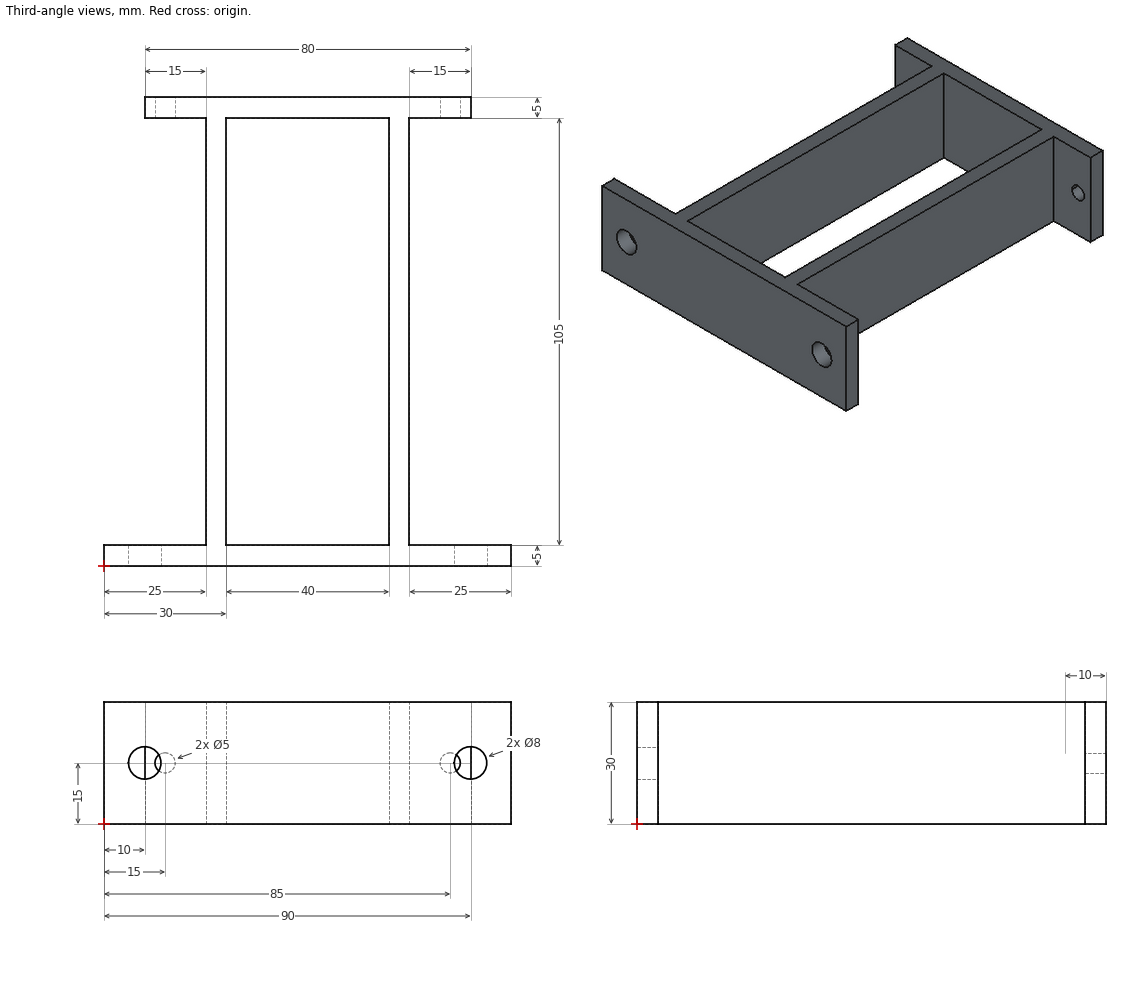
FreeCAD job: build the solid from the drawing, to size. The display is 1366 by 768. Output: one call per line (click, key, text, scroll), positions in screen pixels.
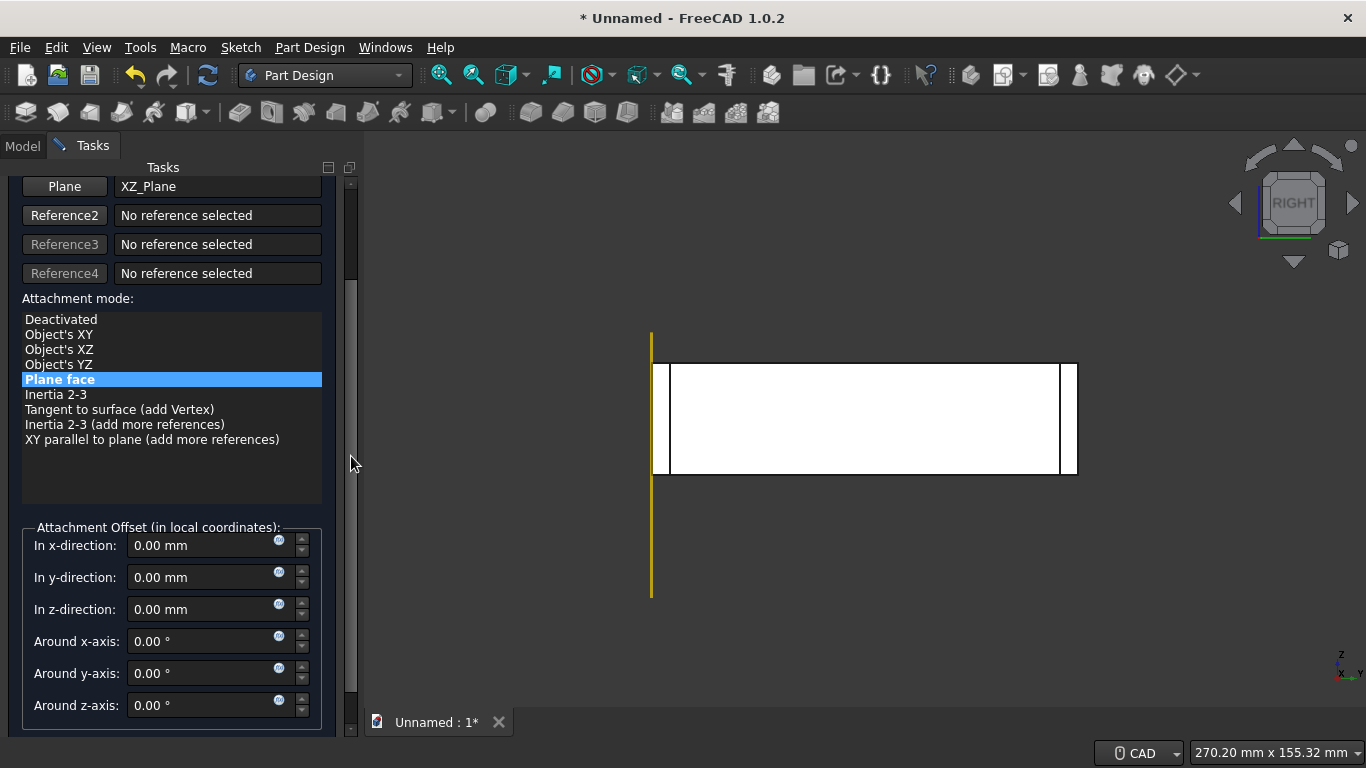
triple_click(210, 609)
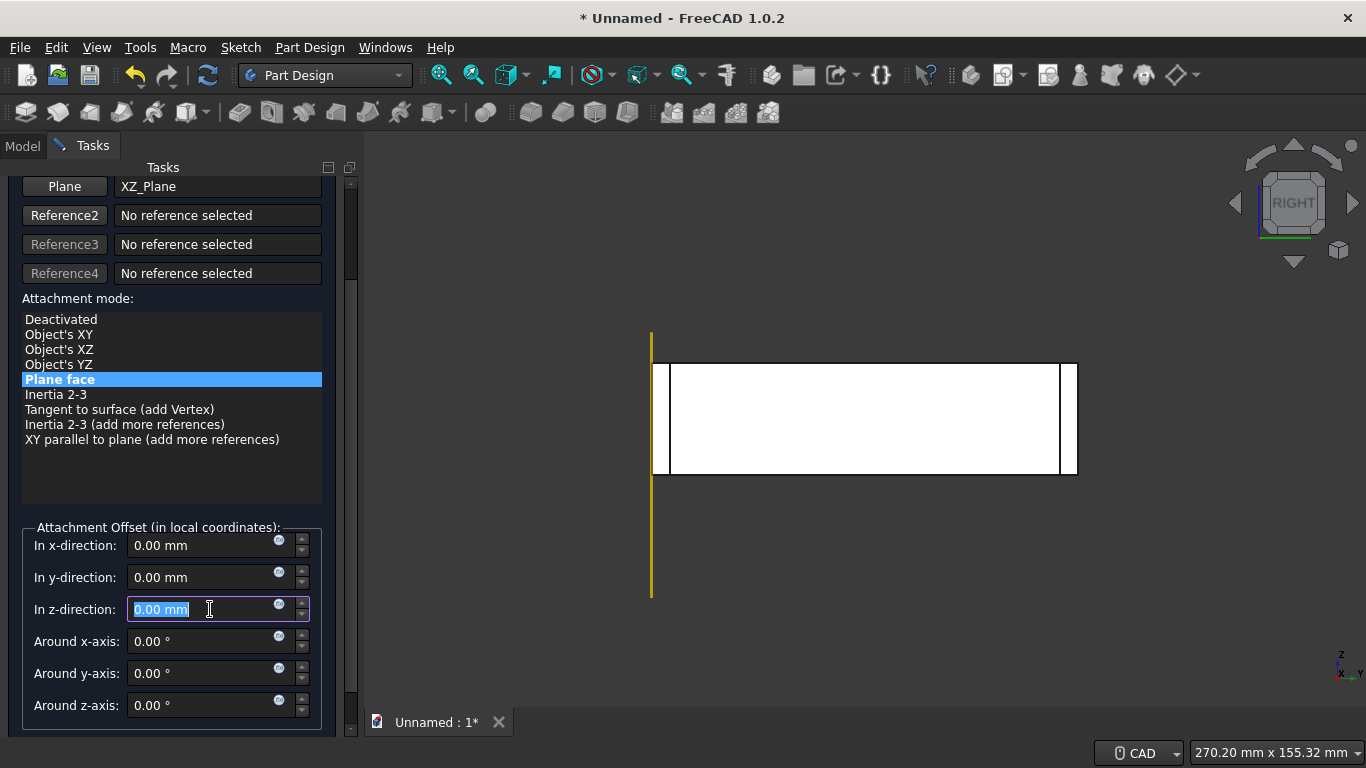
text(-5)
key(Tab)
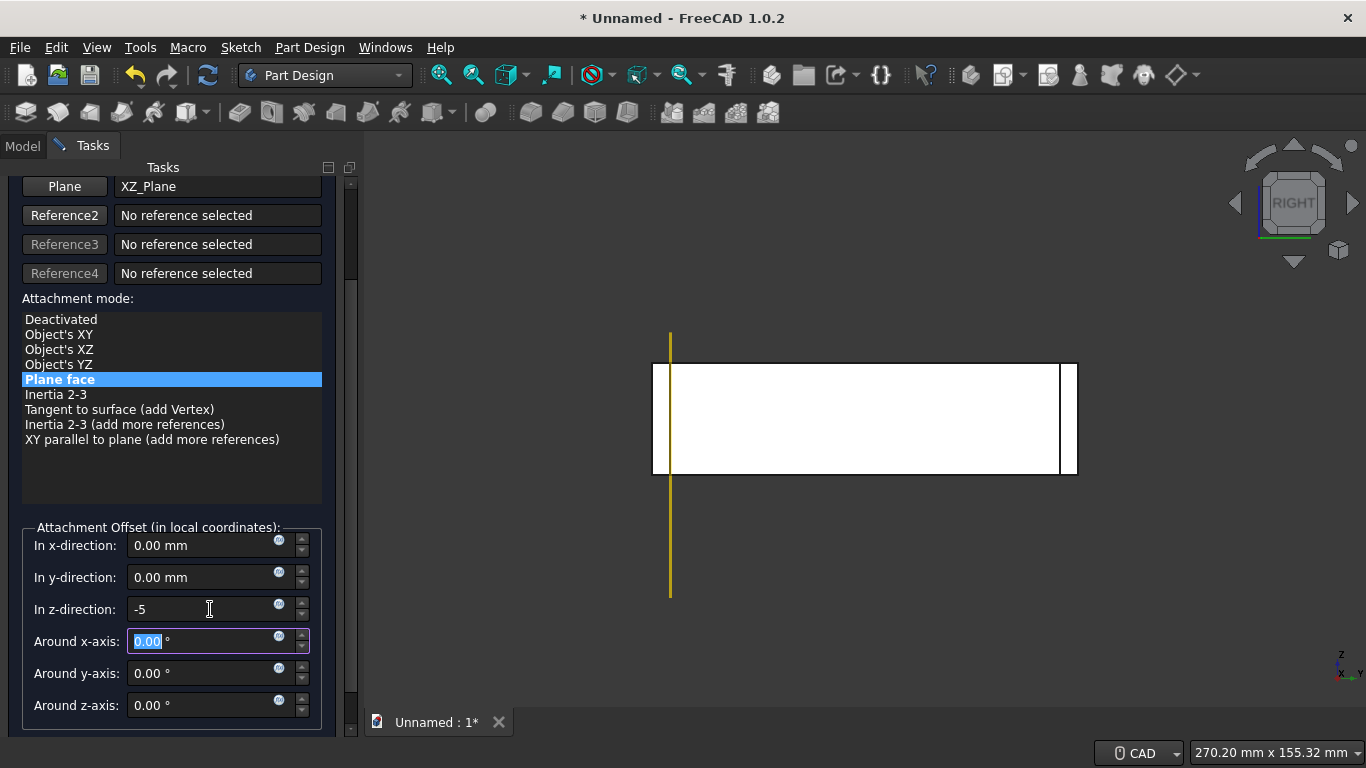
scroll(351, 456, up, 3)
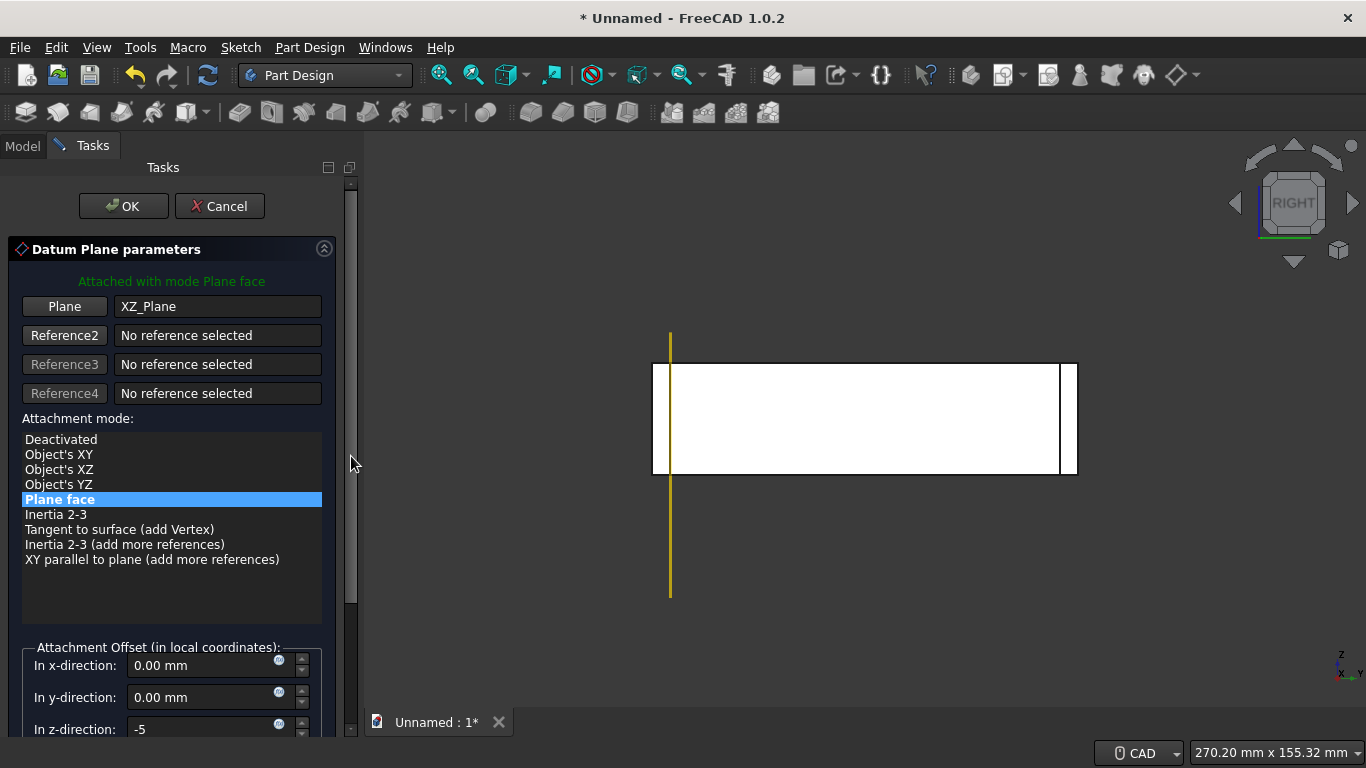
click(124, 206)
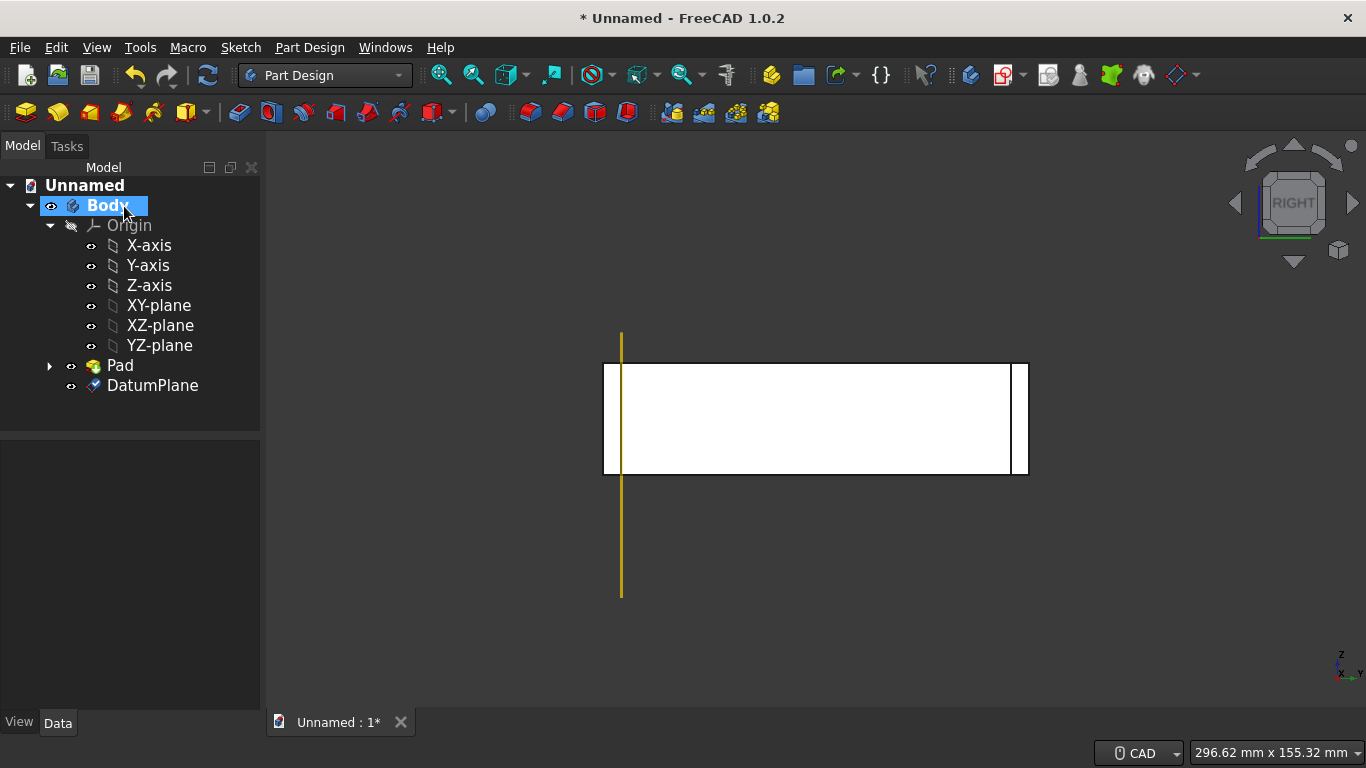
click(116, 386)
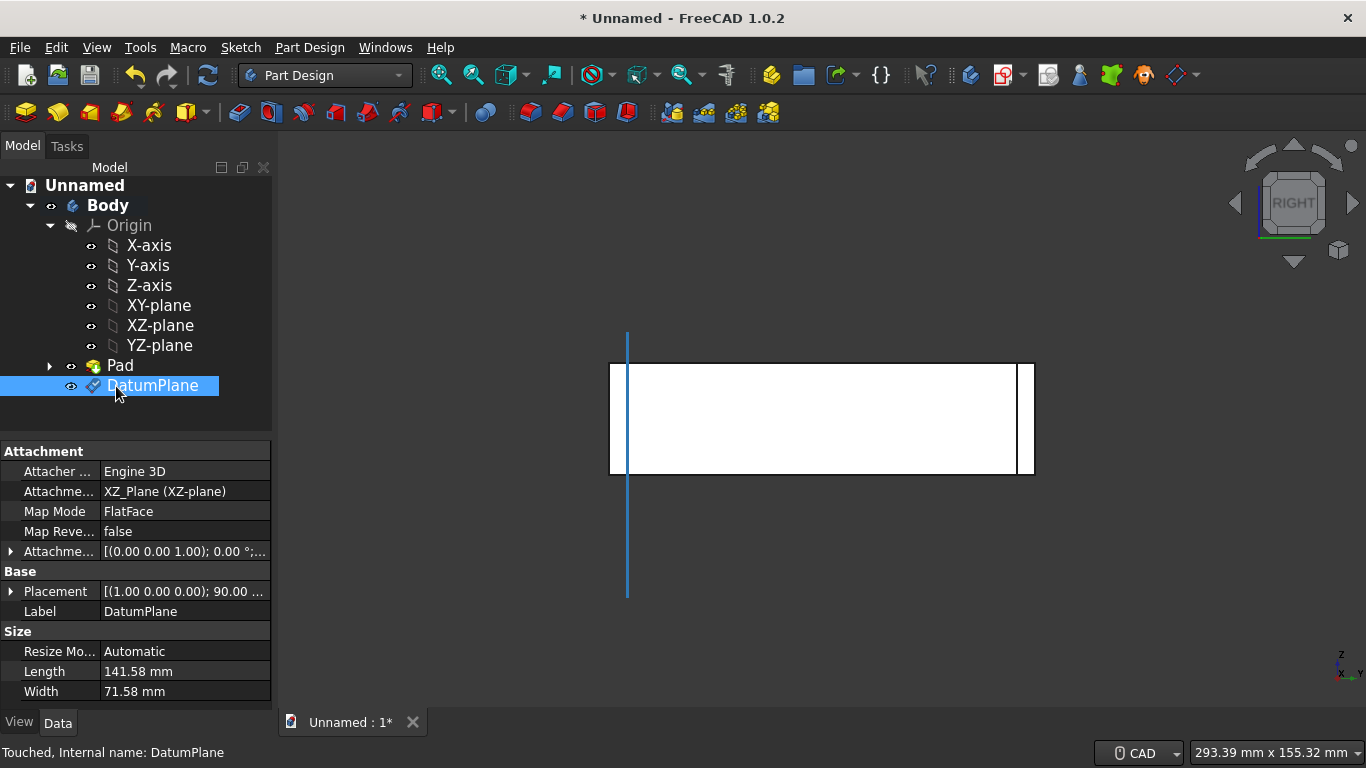
click(1004, 76)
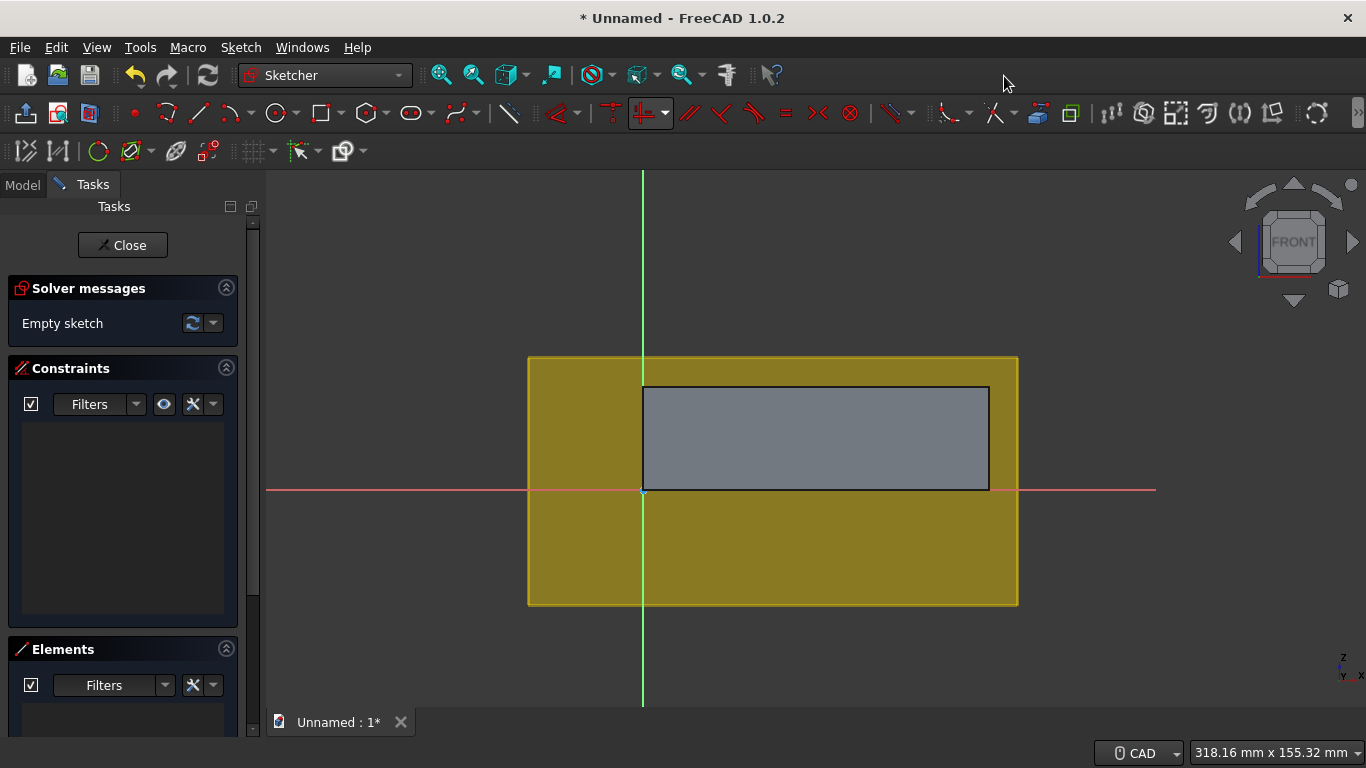
click(90, 114)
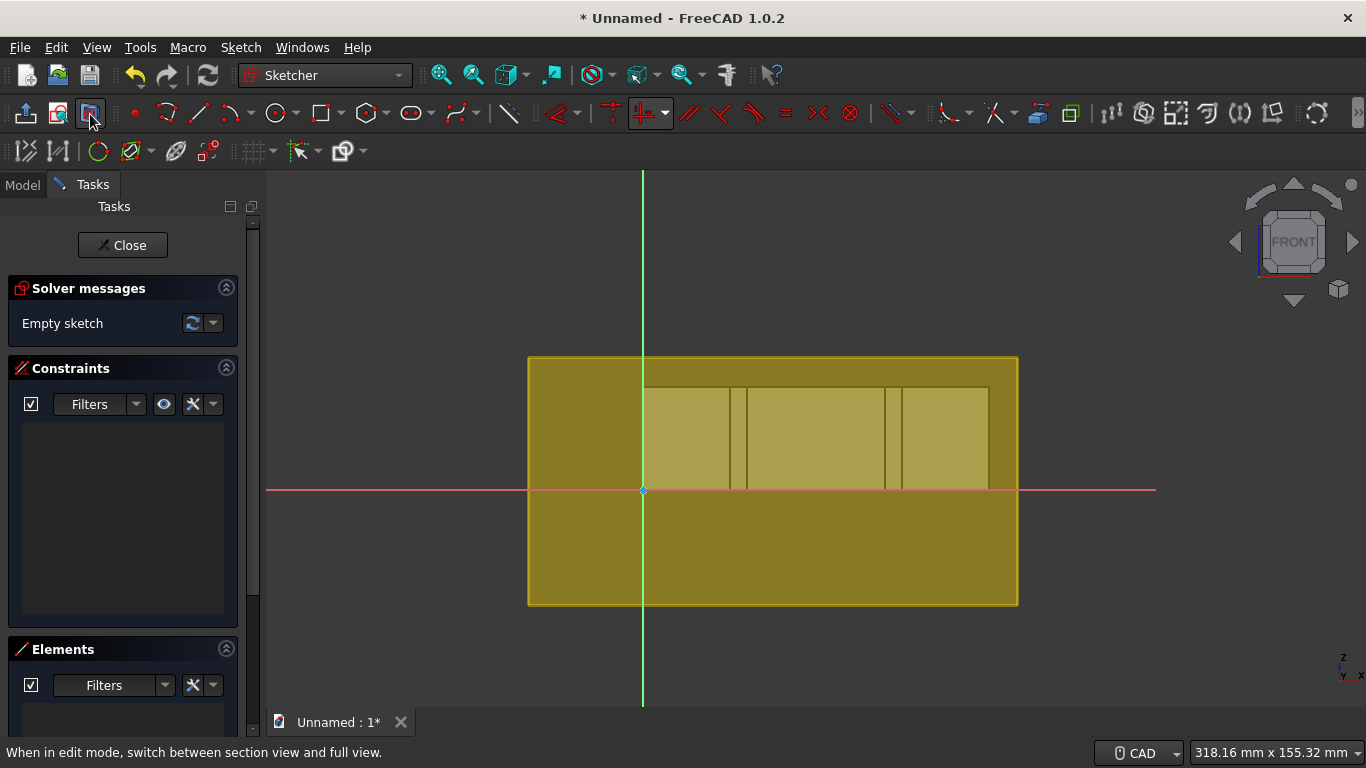
scroll(876, 481, up, 3)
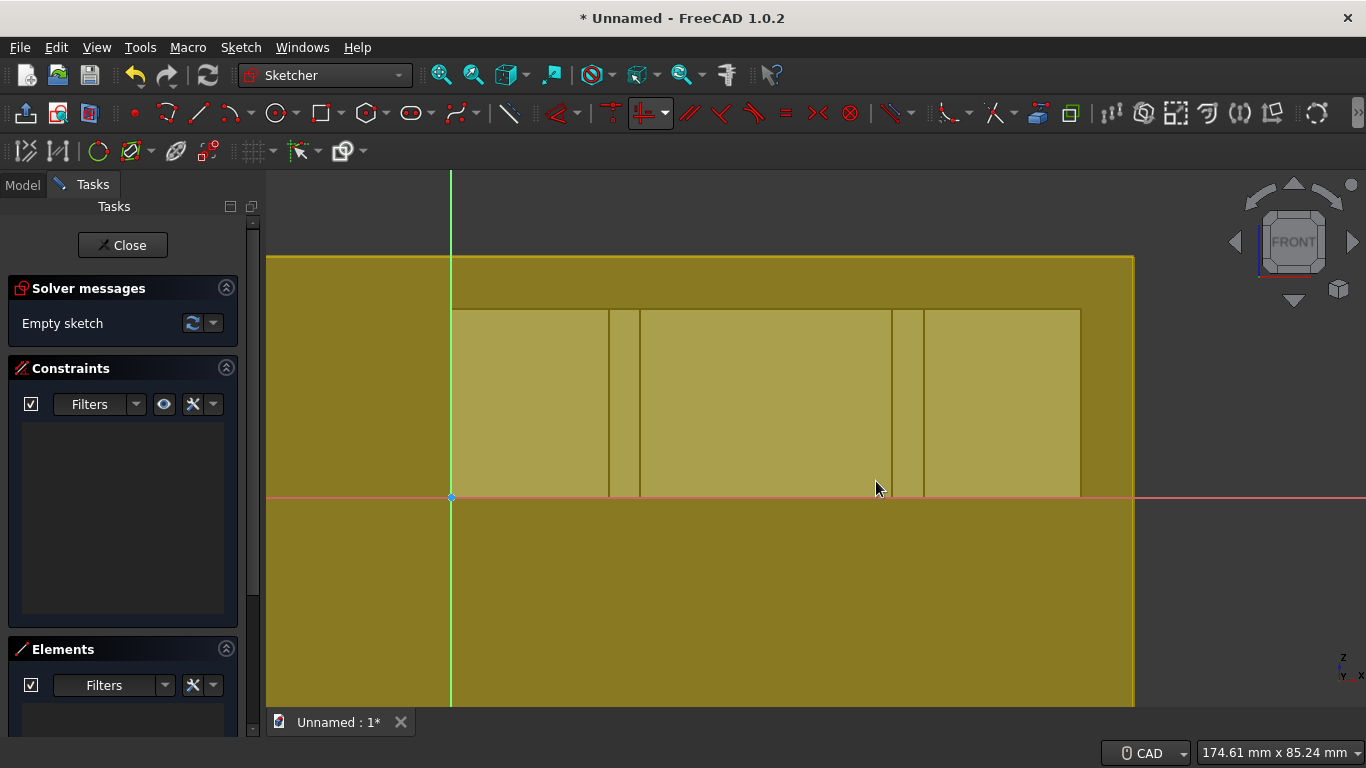
click(276, 114)